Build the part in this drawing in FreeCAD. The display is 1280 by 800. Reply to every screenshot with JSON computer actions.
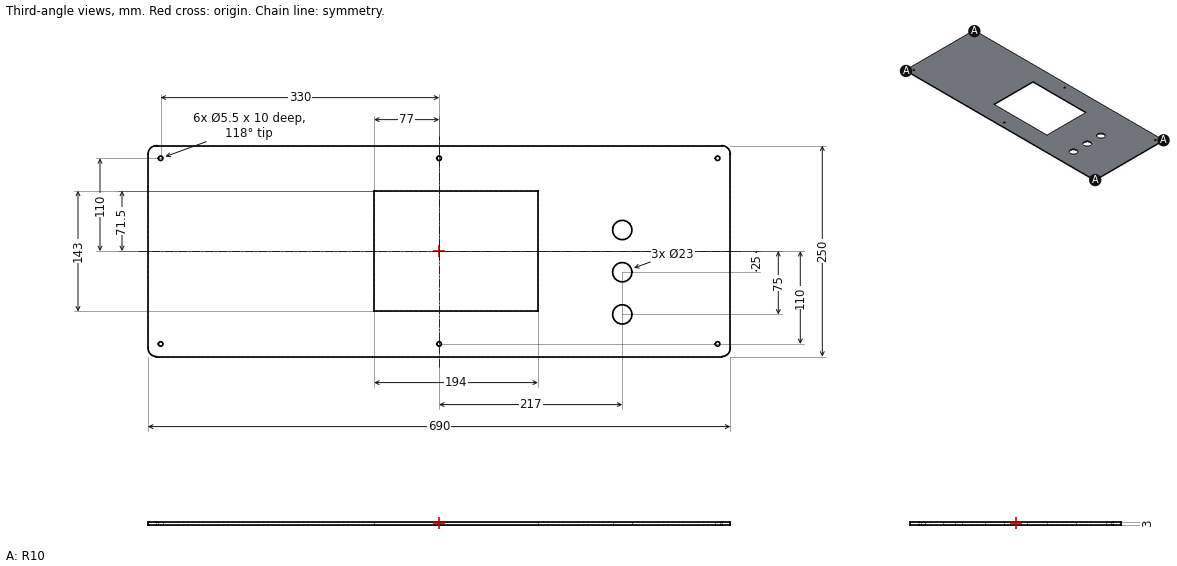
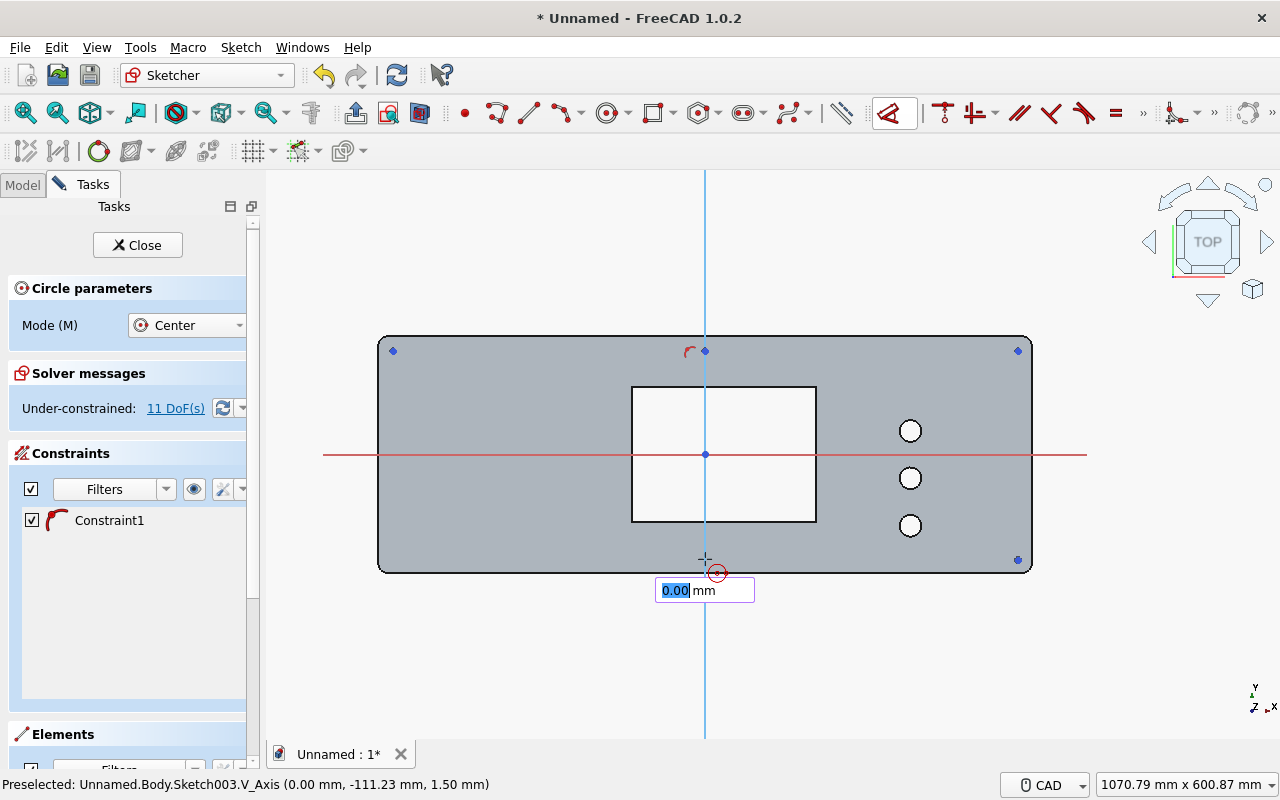
{"action": "scroll", "coordinate": [707, 558], "scroll_direction": "up", "scroll_amount": 10}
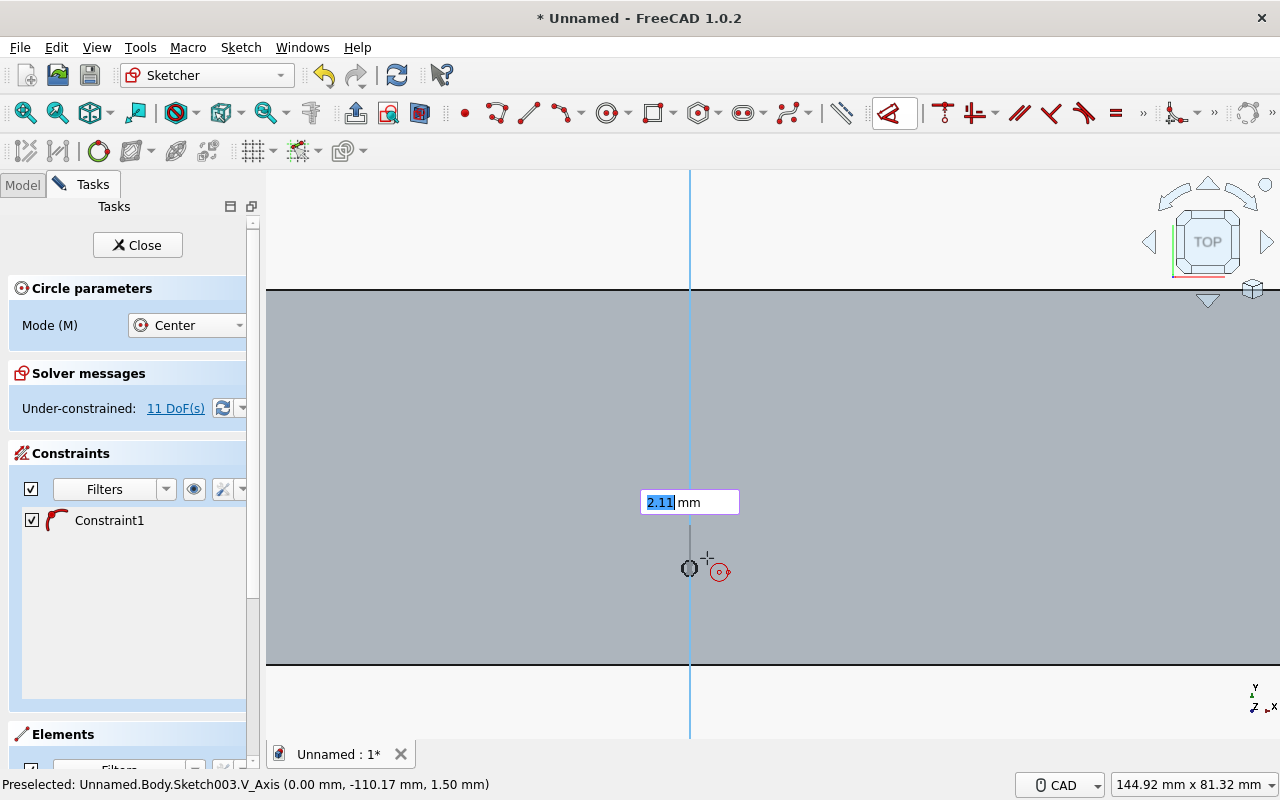
{"action": "left_click", "coordinate": [708, 553]}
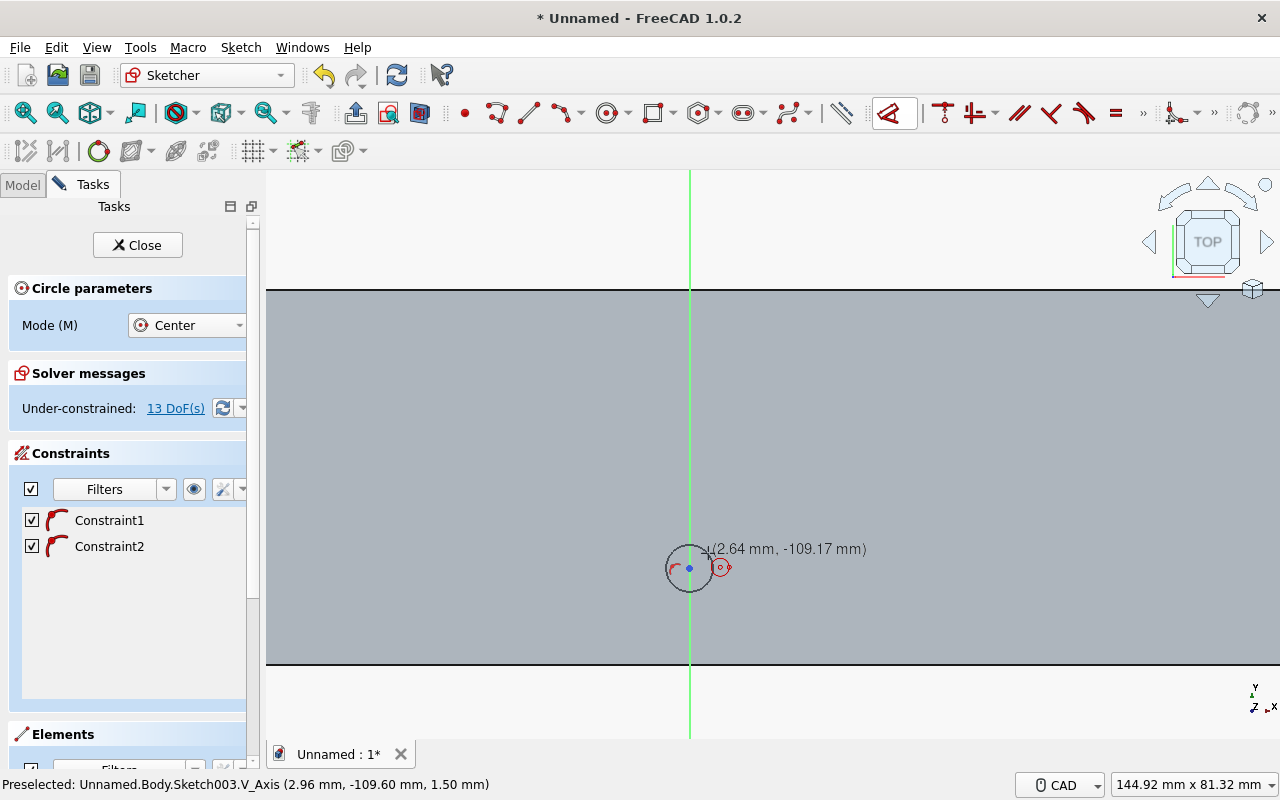
{"action": "scroll", "coordinate": [707, 558], "scroll_direction": "down", "scroll_amount": 10}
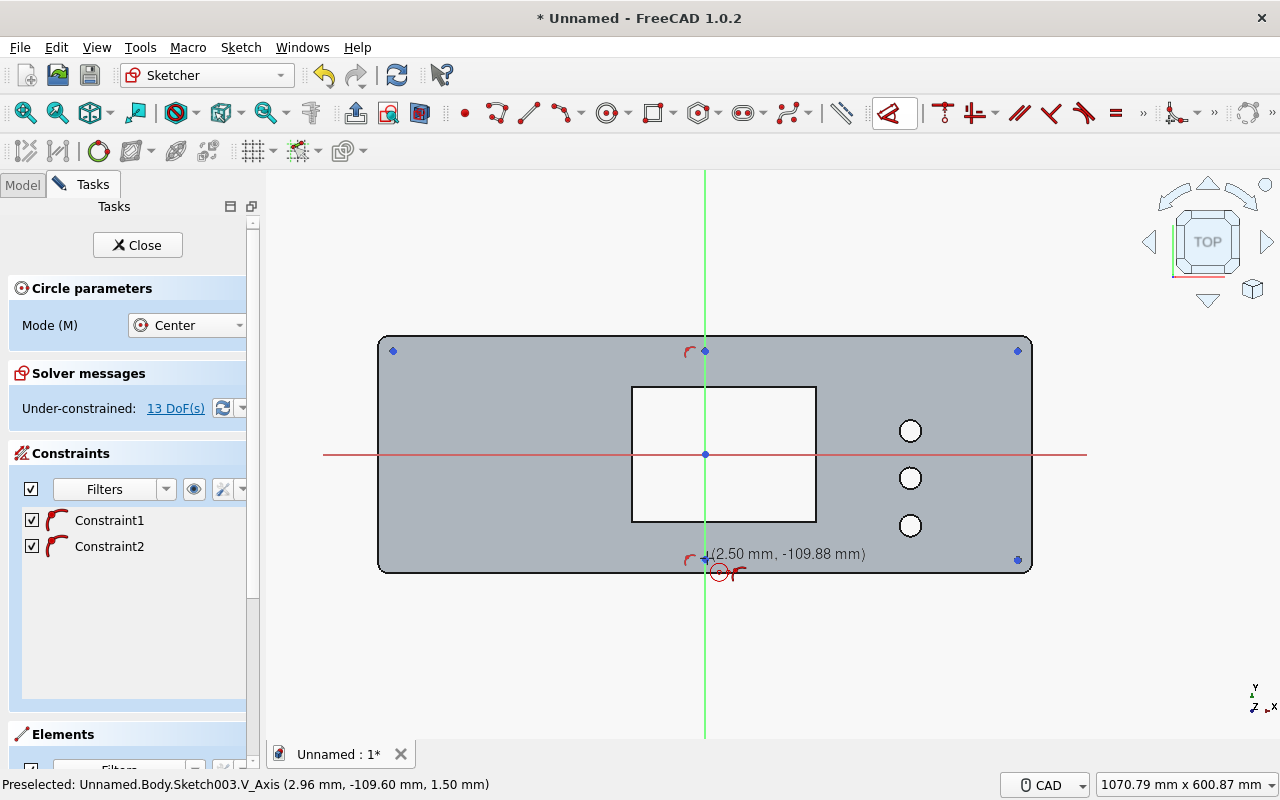
{"action": "scroll", "coordinate": [393, 559], "scroll_direction": "up", "scroll_amount": 11}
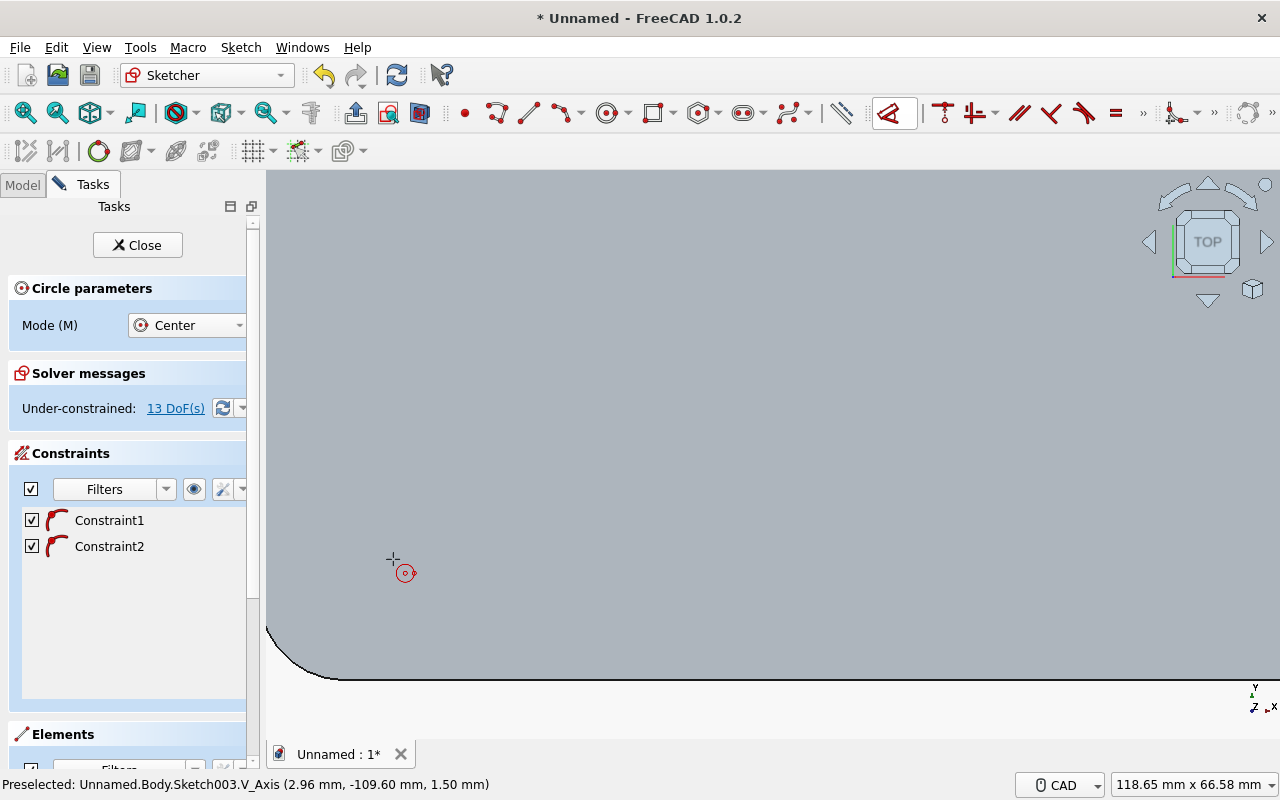
{"action": "scroll", "coordinate": [393, 559], "scroll_direction": "down", "scroll_amount": 11}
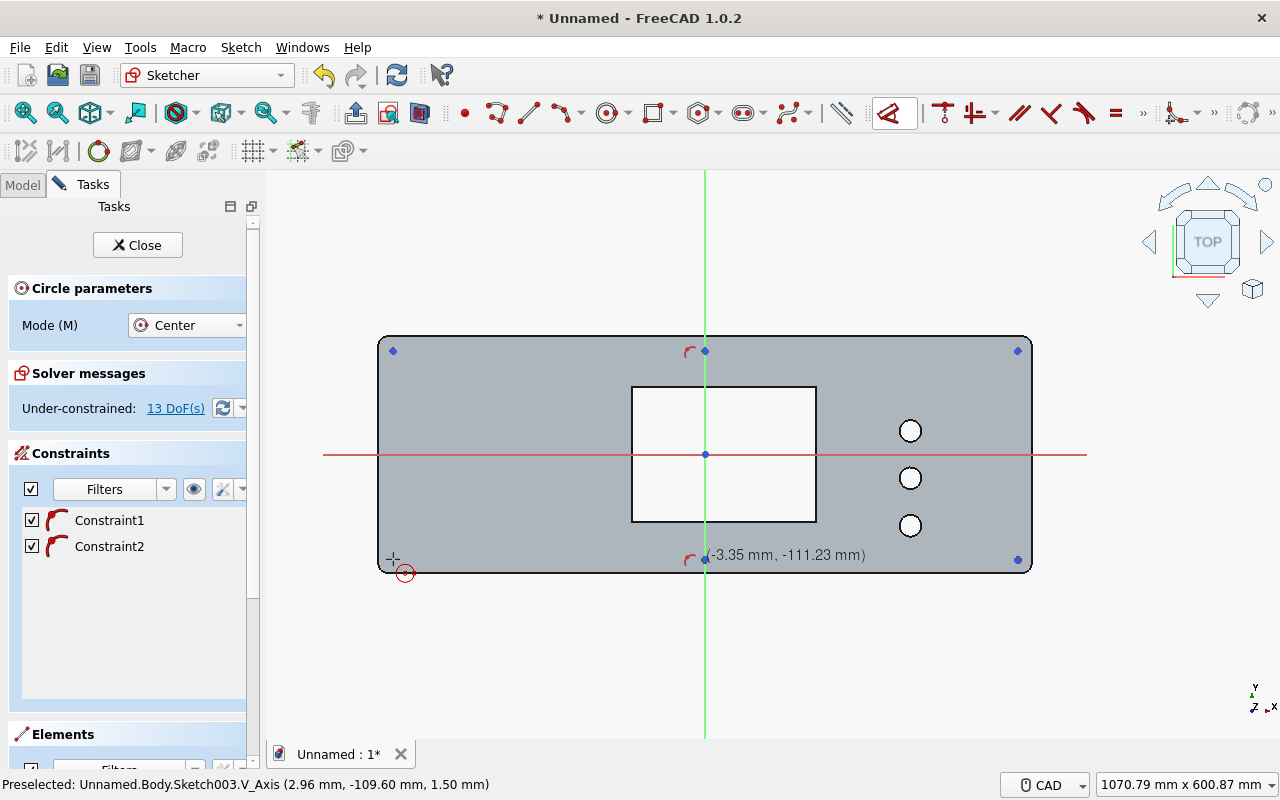
{"action": "left_click", "coordinate": [393, 559]}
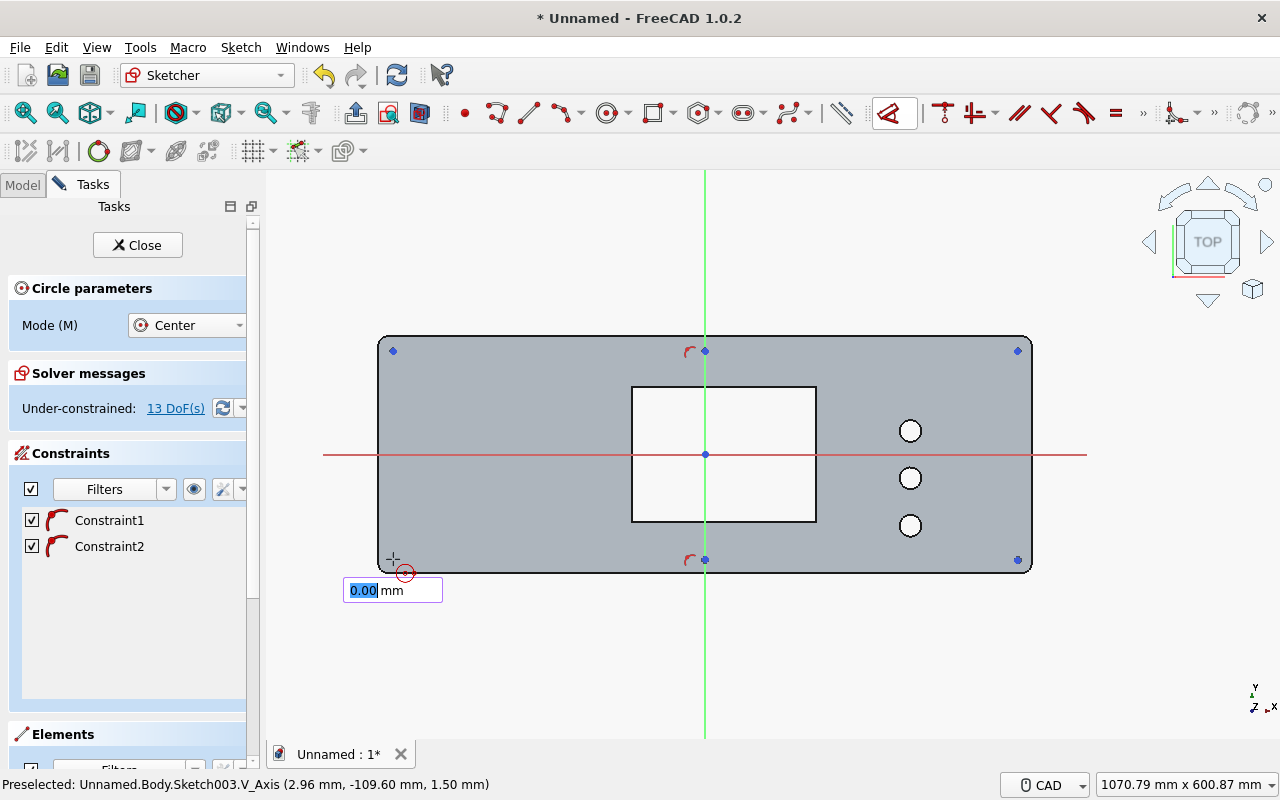
{"action": "scroll", "coordinate": [394, 557], "scroll_direction": "up", "scroll_amount": 10}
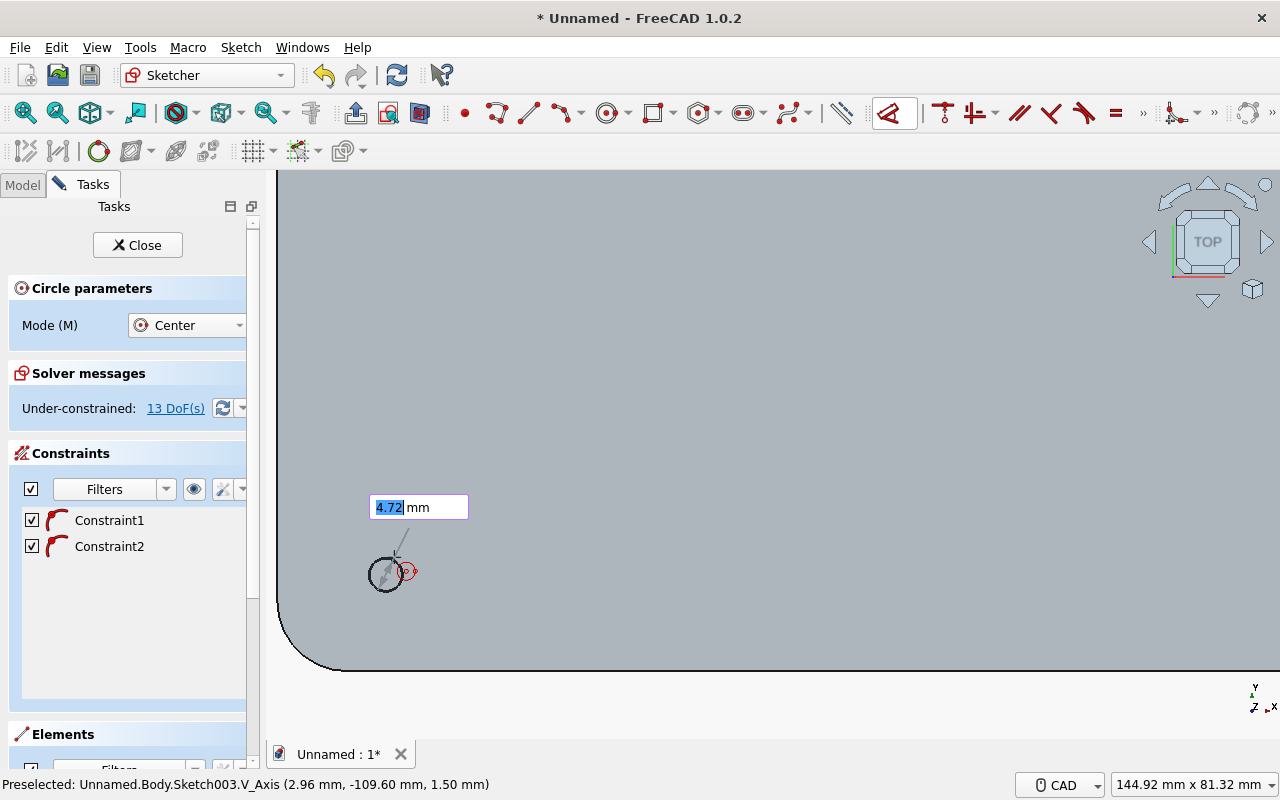
{"action": "left_click", "coordinate": [396, 553]}
{"action": "key", "text": "Escape"}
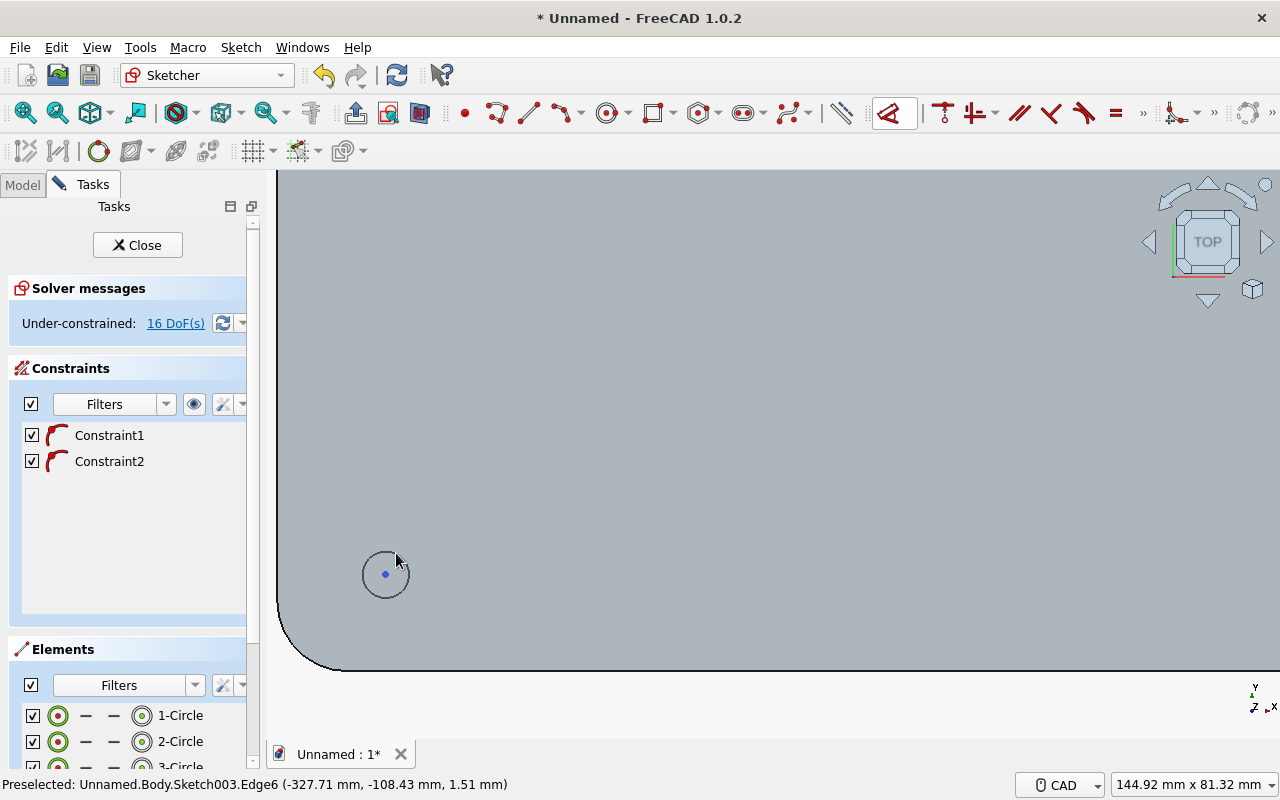
{"action": "scroll", "coordinate": [394, 557], "scroll_direction": "down", "scroll_amount": 10}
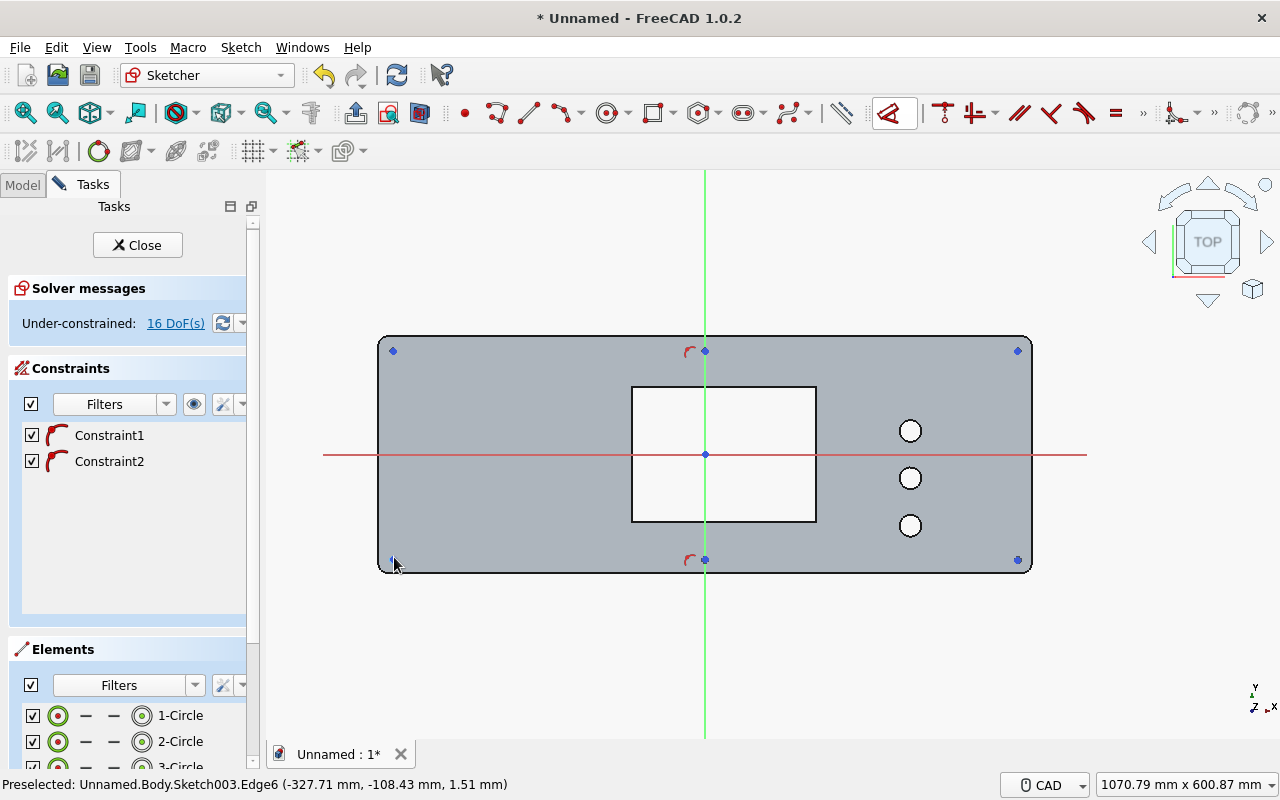
{"action": "scroll", "coordinate": [395, 349], "scroll_direction": "up", "scroll_amount": 9}